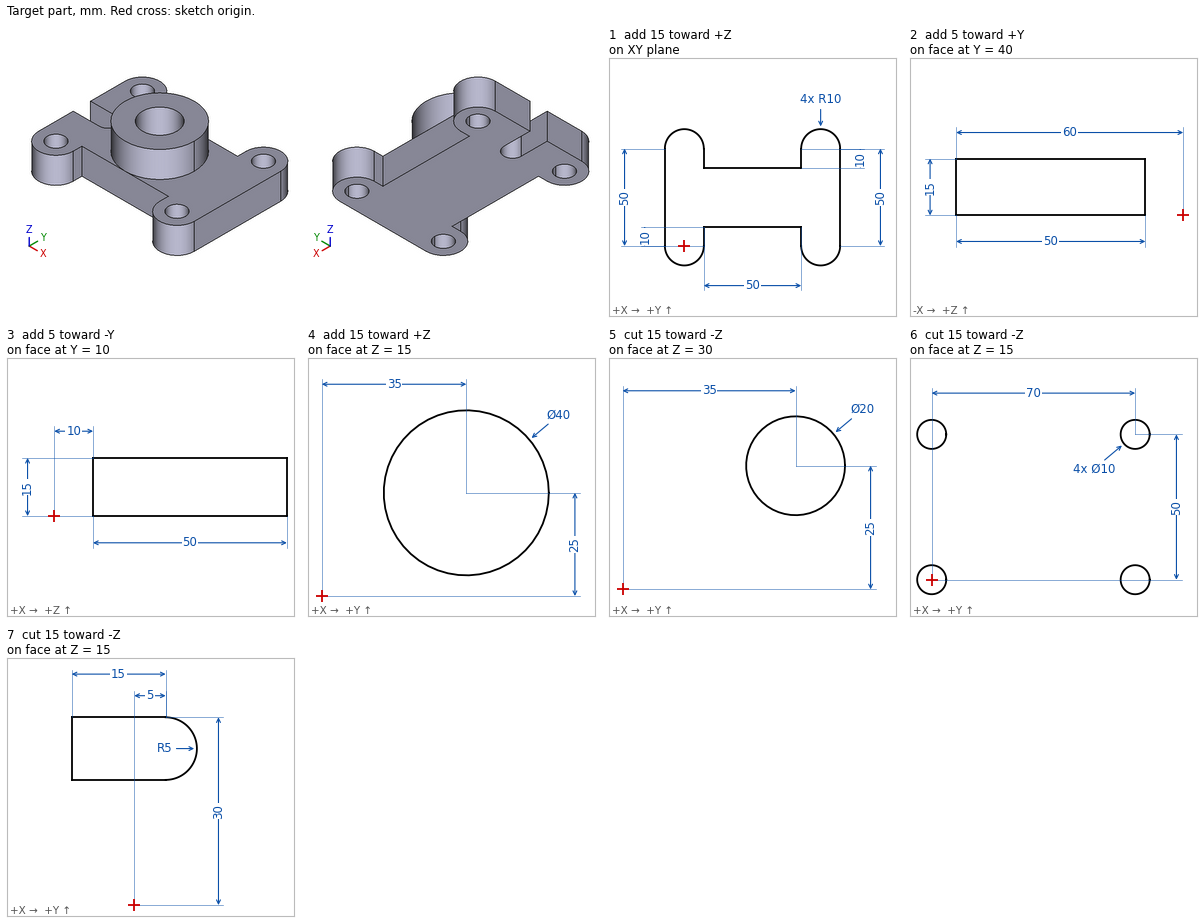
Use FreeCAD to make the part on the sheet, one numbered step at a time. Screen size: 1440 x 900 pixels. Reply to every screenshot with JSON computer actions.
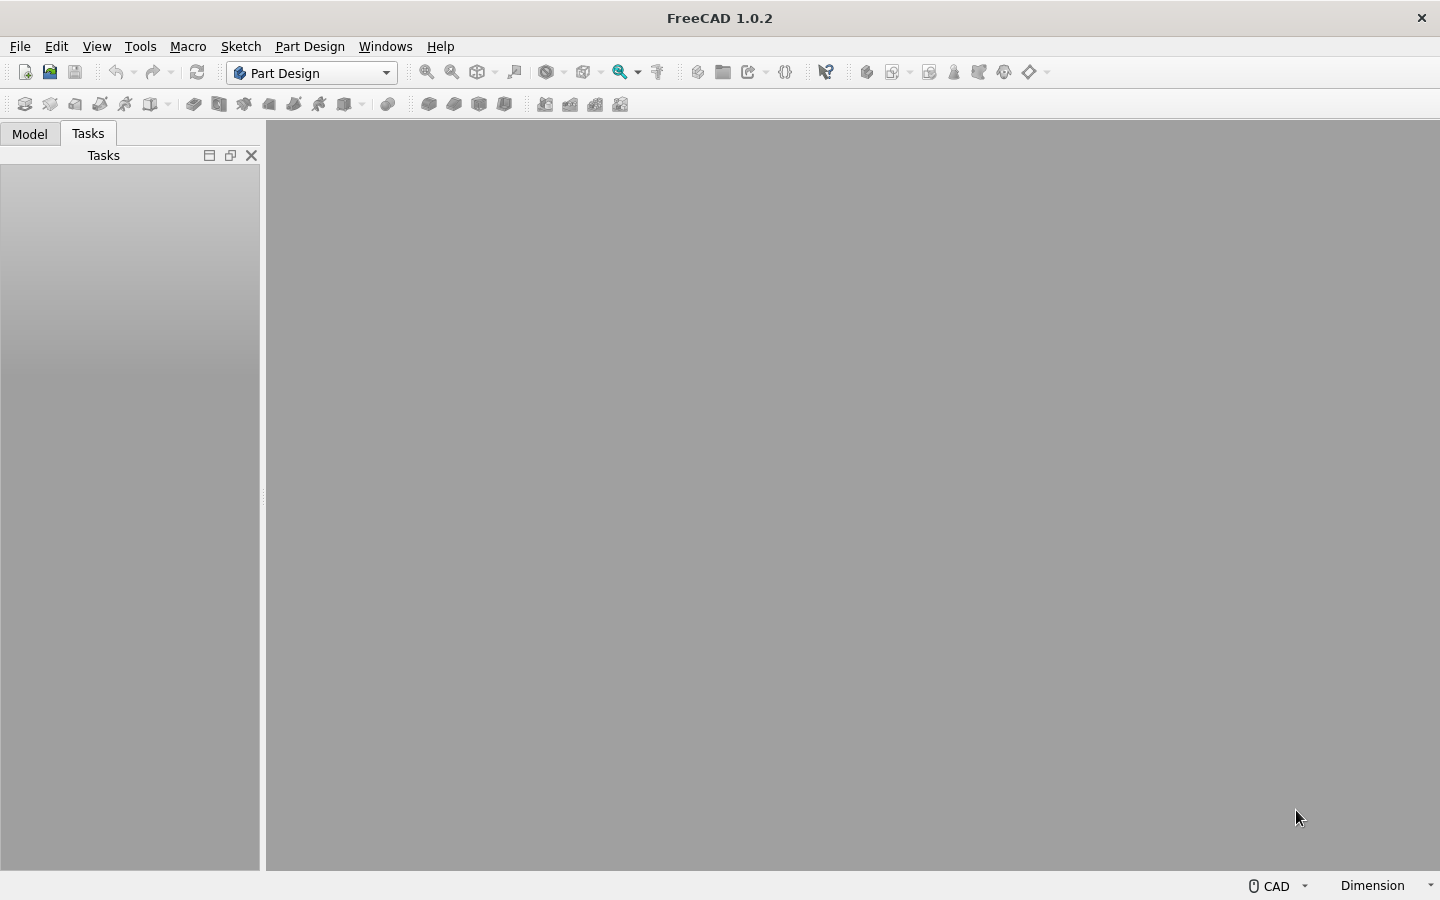
{"action": "left_click", "coordinate": [25, 72]}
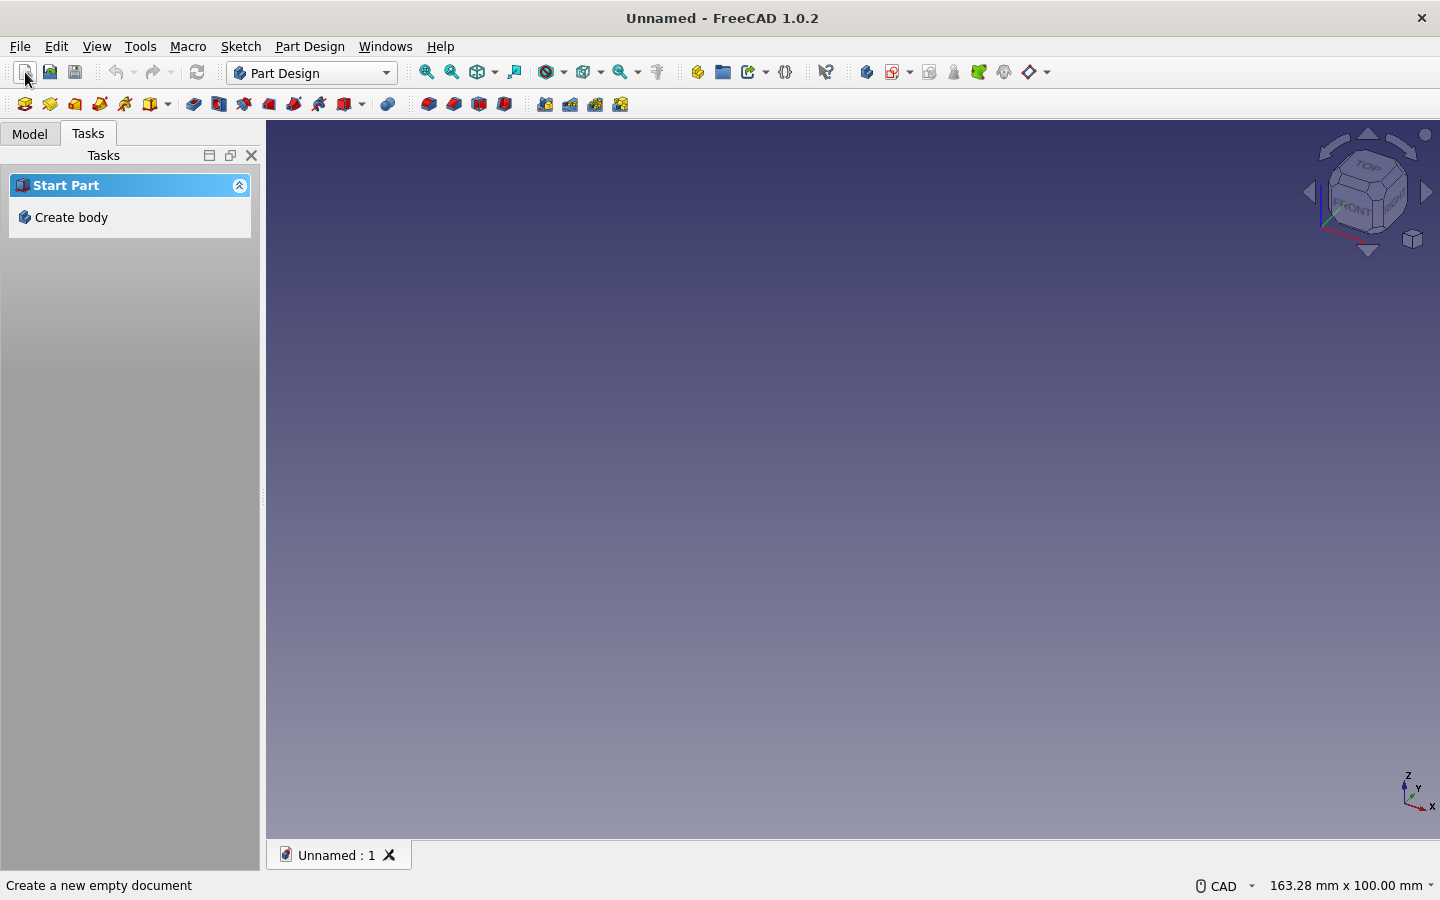
{"action": "left_click", "coordinate": [892, 72]}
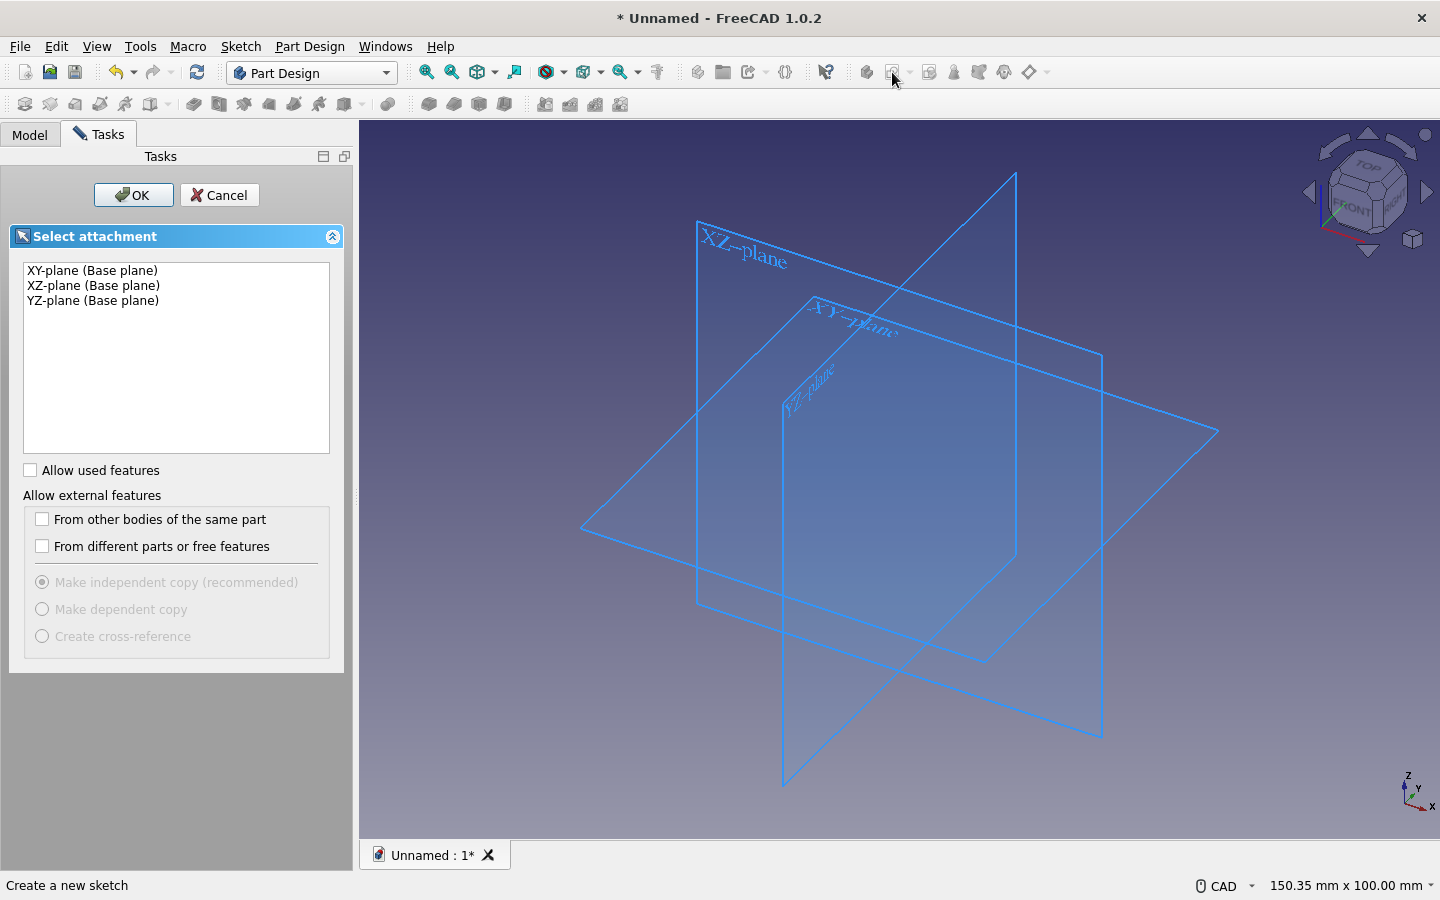
{"action": "left_click", "coordinate": [84, 270]}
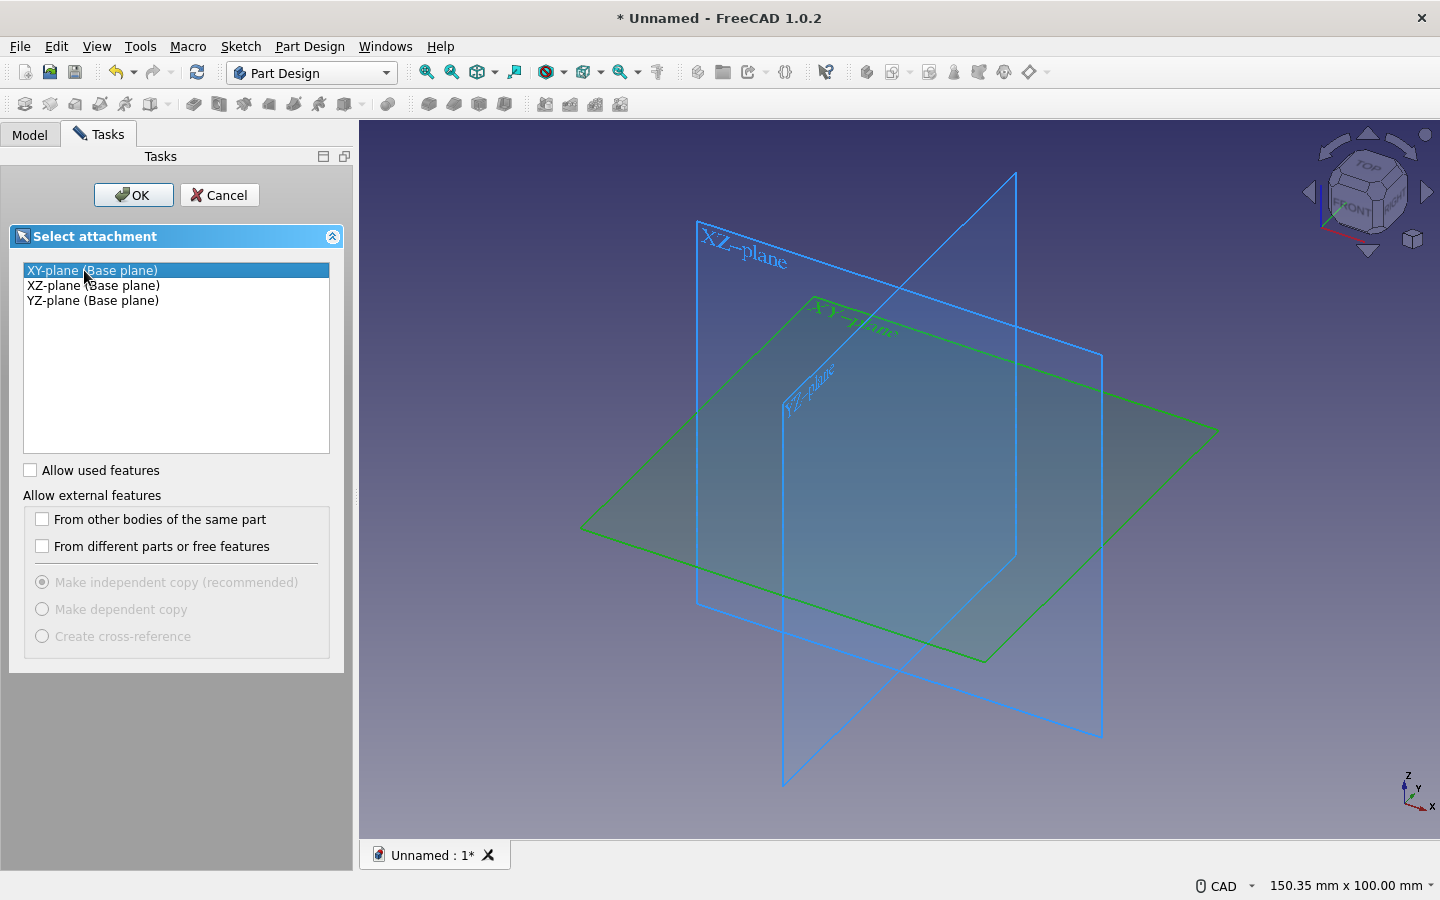
{"action": "left_click", "coordinate": [134, 195]}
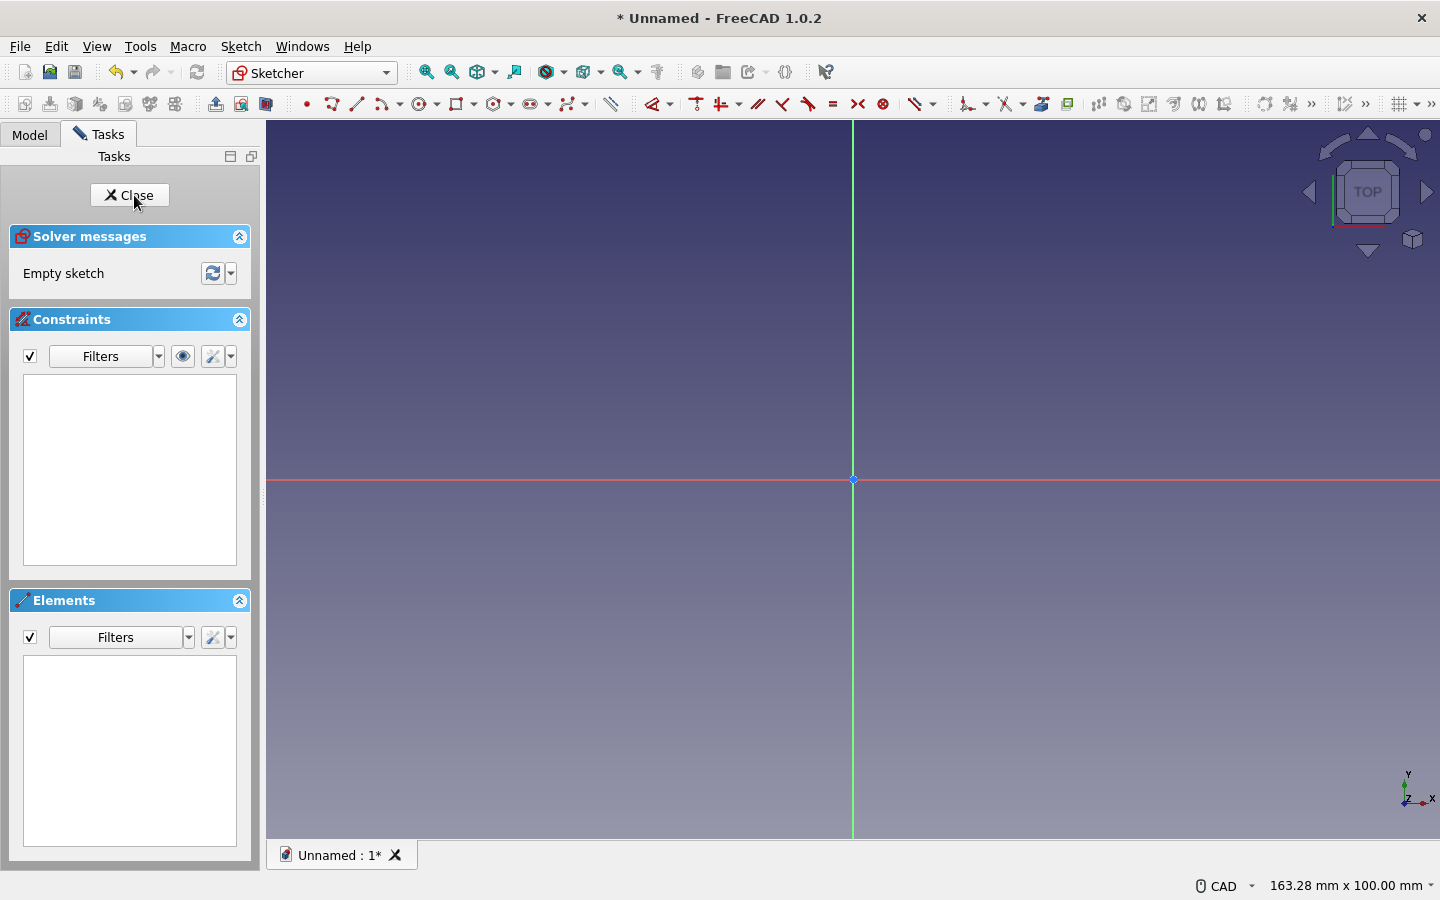
{"action": "scroll", "coordinate": [294, 811], "scroll_direction": "down", "scroll_amount": 1}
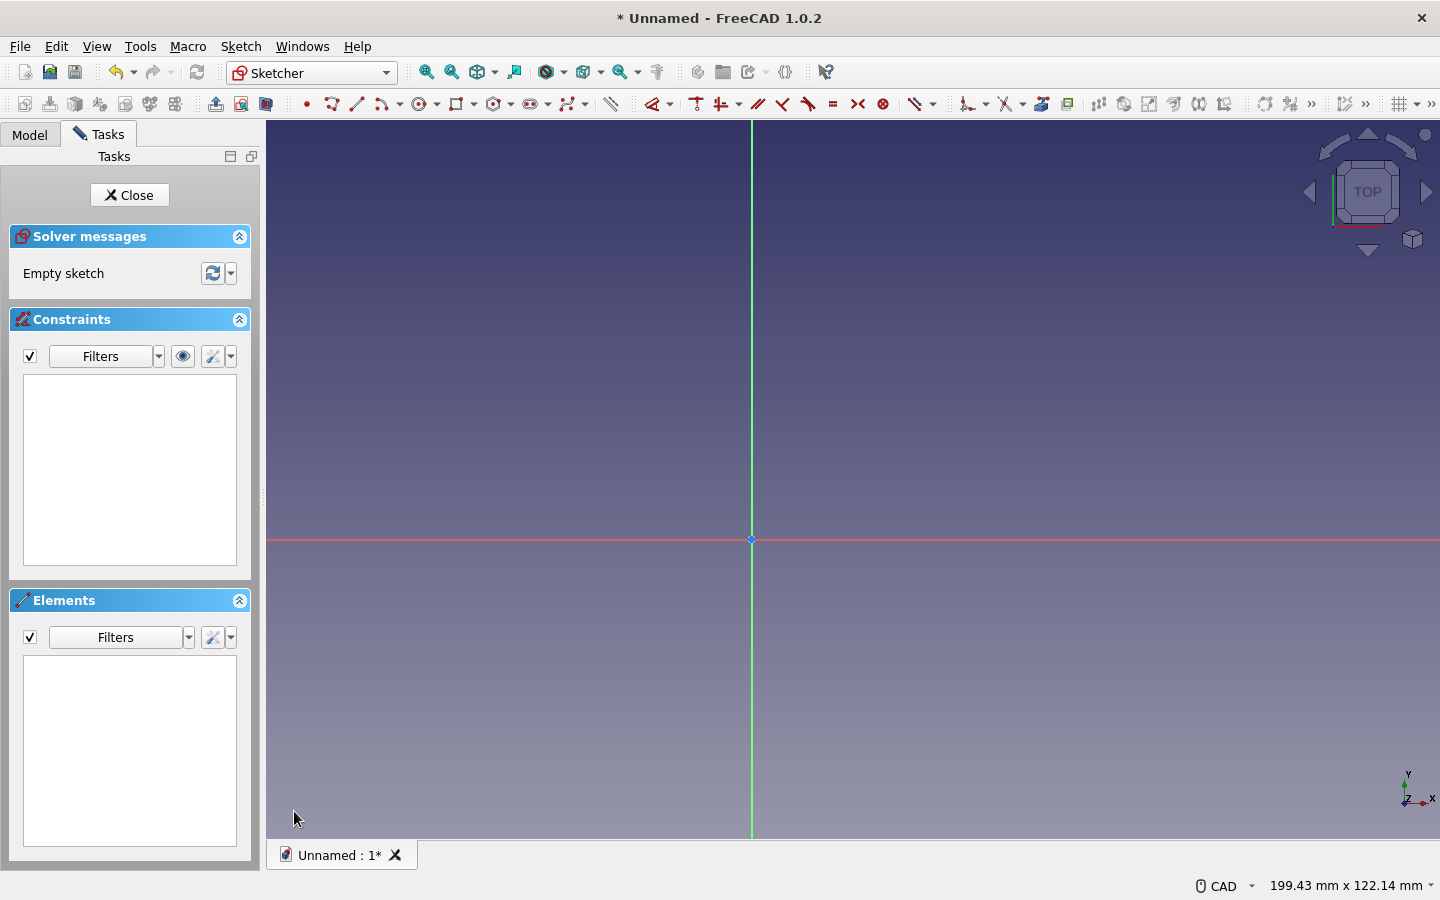
{"action": "left_click", "coordinate": [357, 104]}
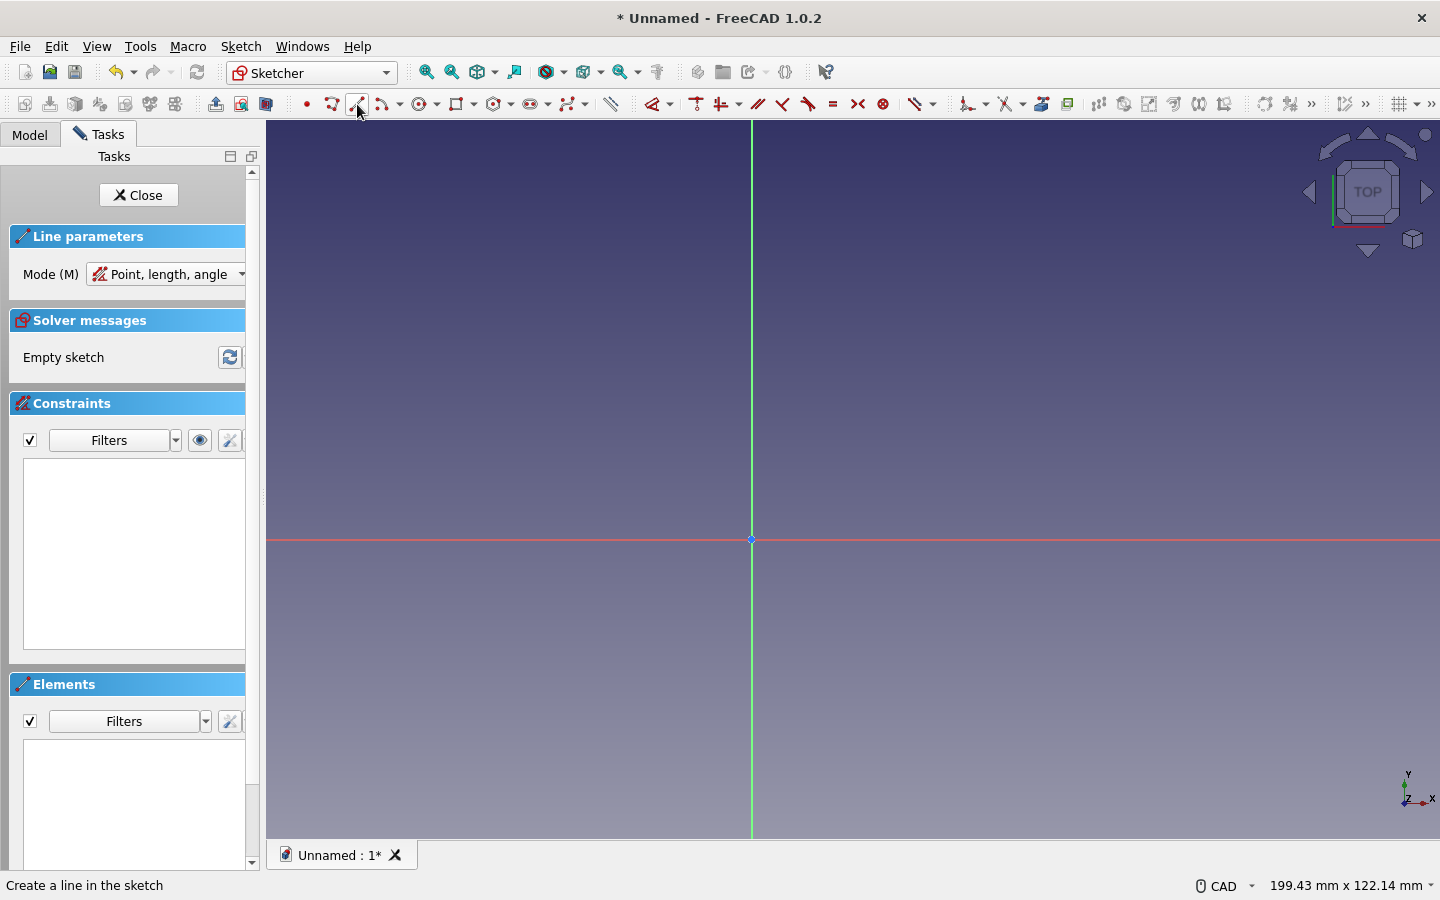
{"action": "left_click", "coordinate": [693, 245]}
{"action": "left_click", "coordinate": [693, 540]}